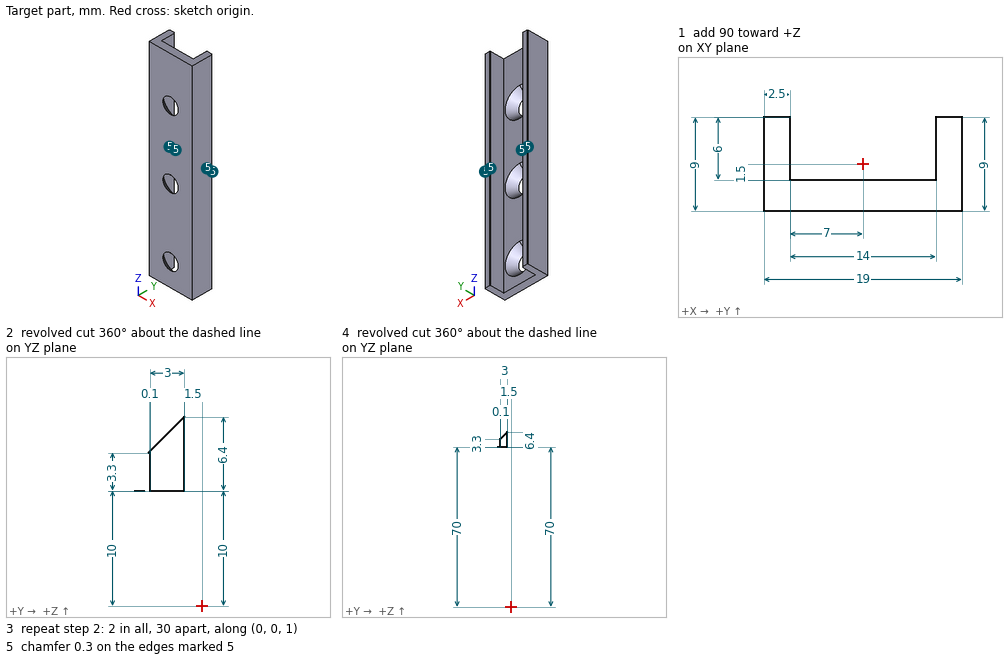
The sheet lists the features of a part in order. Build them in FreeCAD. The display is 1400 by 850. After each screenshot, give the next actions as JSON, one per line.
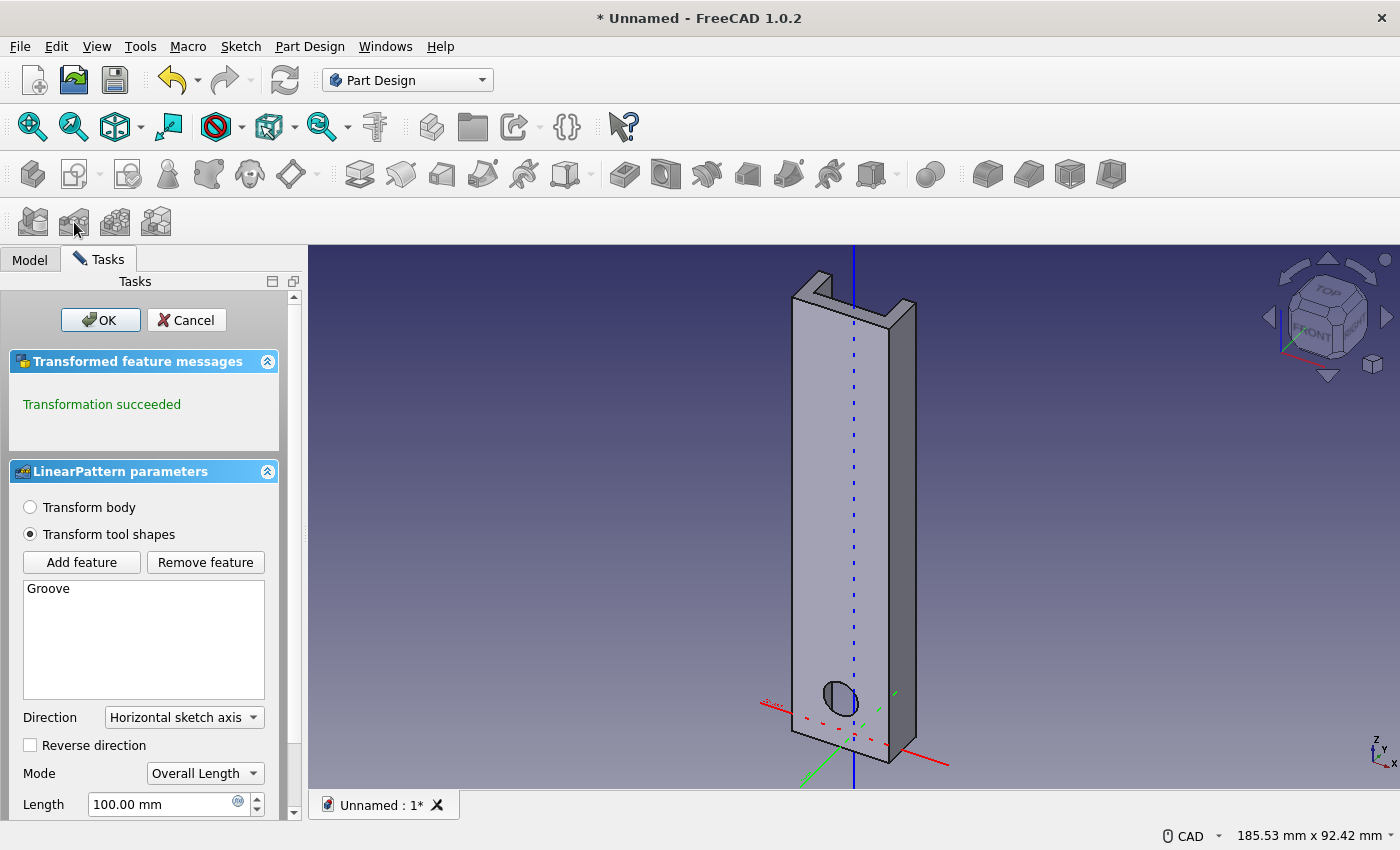
{"action": "left_click", "coordinate": [185, 718]}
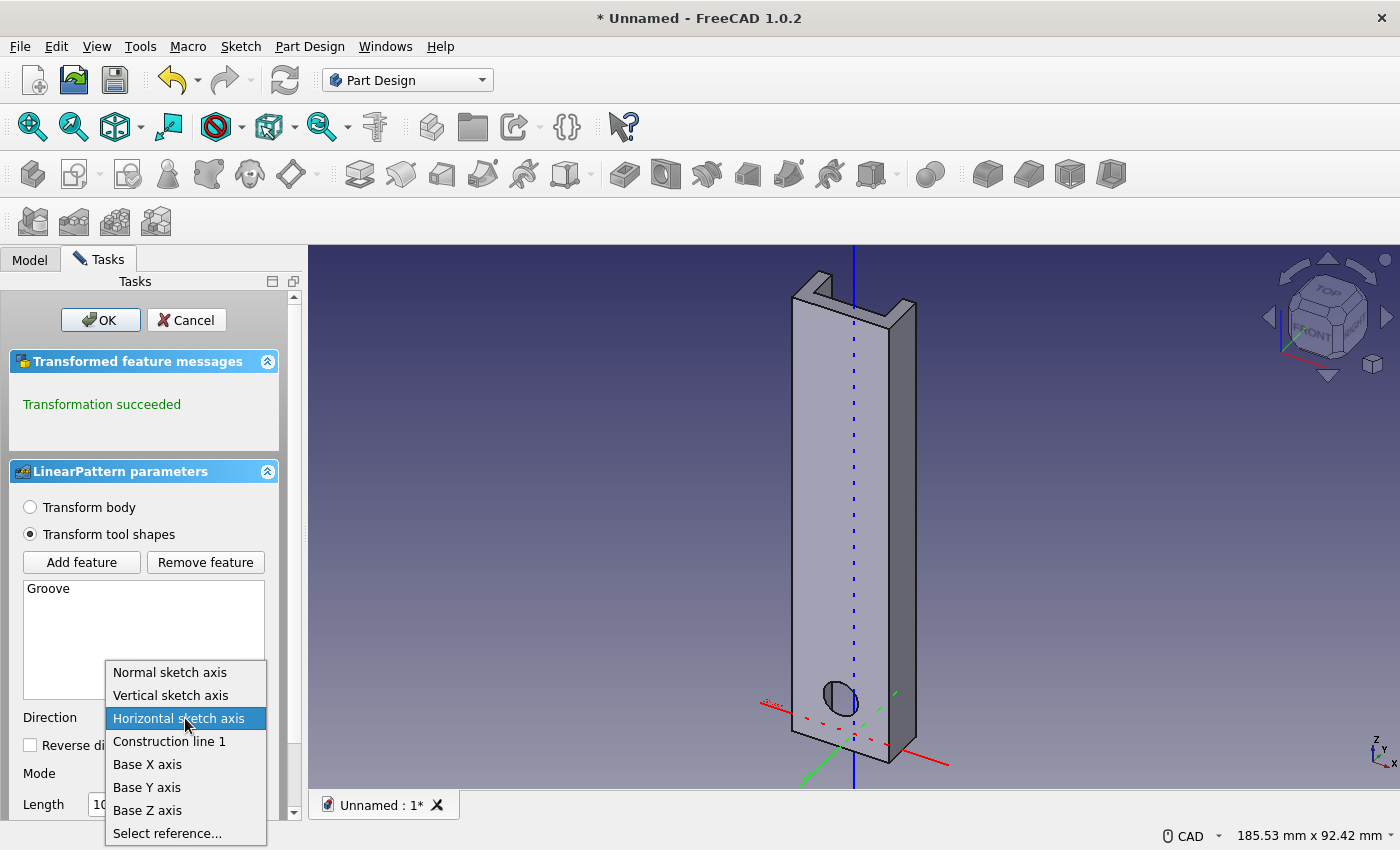
{"action": "left_click", "coordinate": [184, 810]}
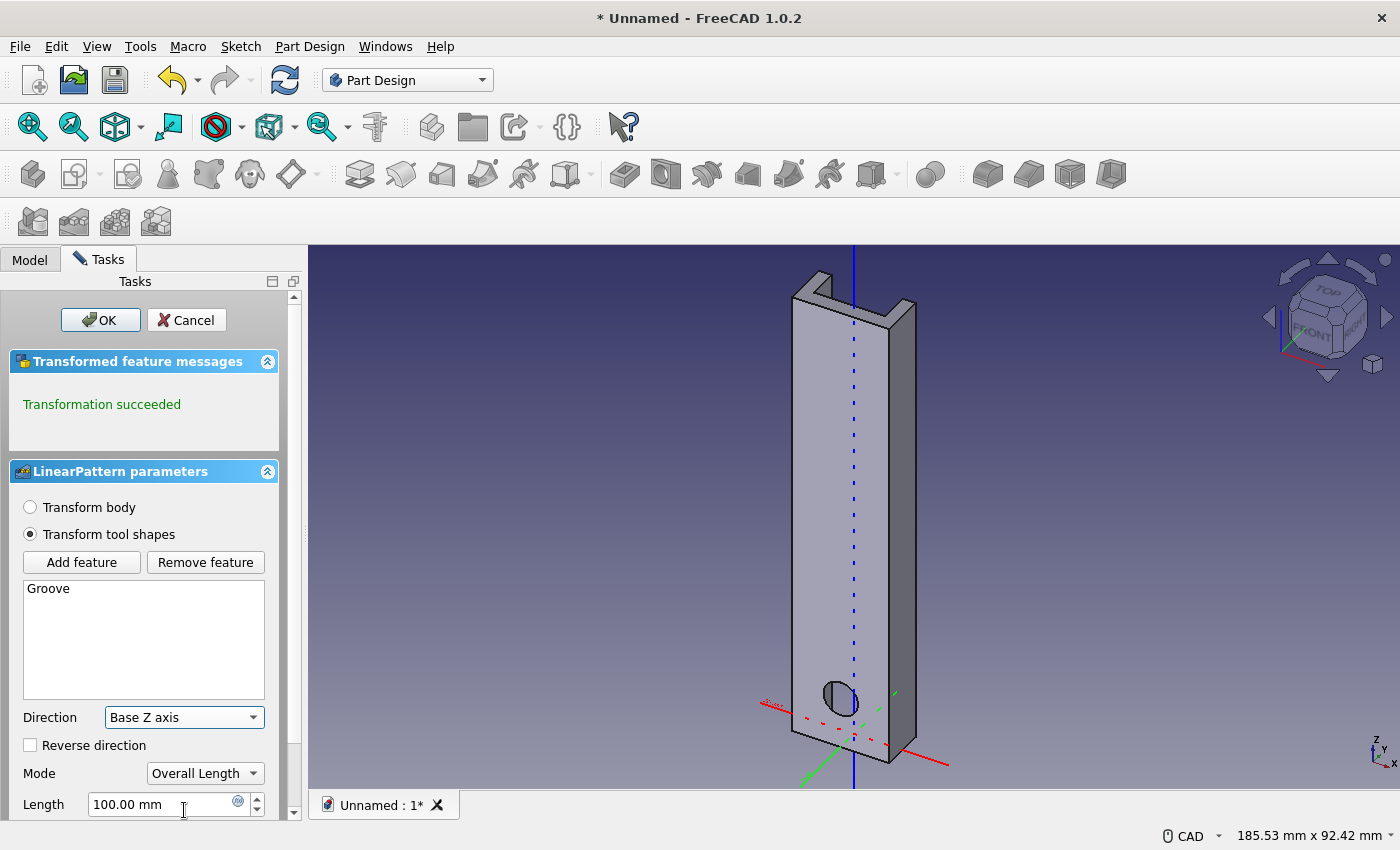
{"action": "left_click", "coordinate": [206, 774]}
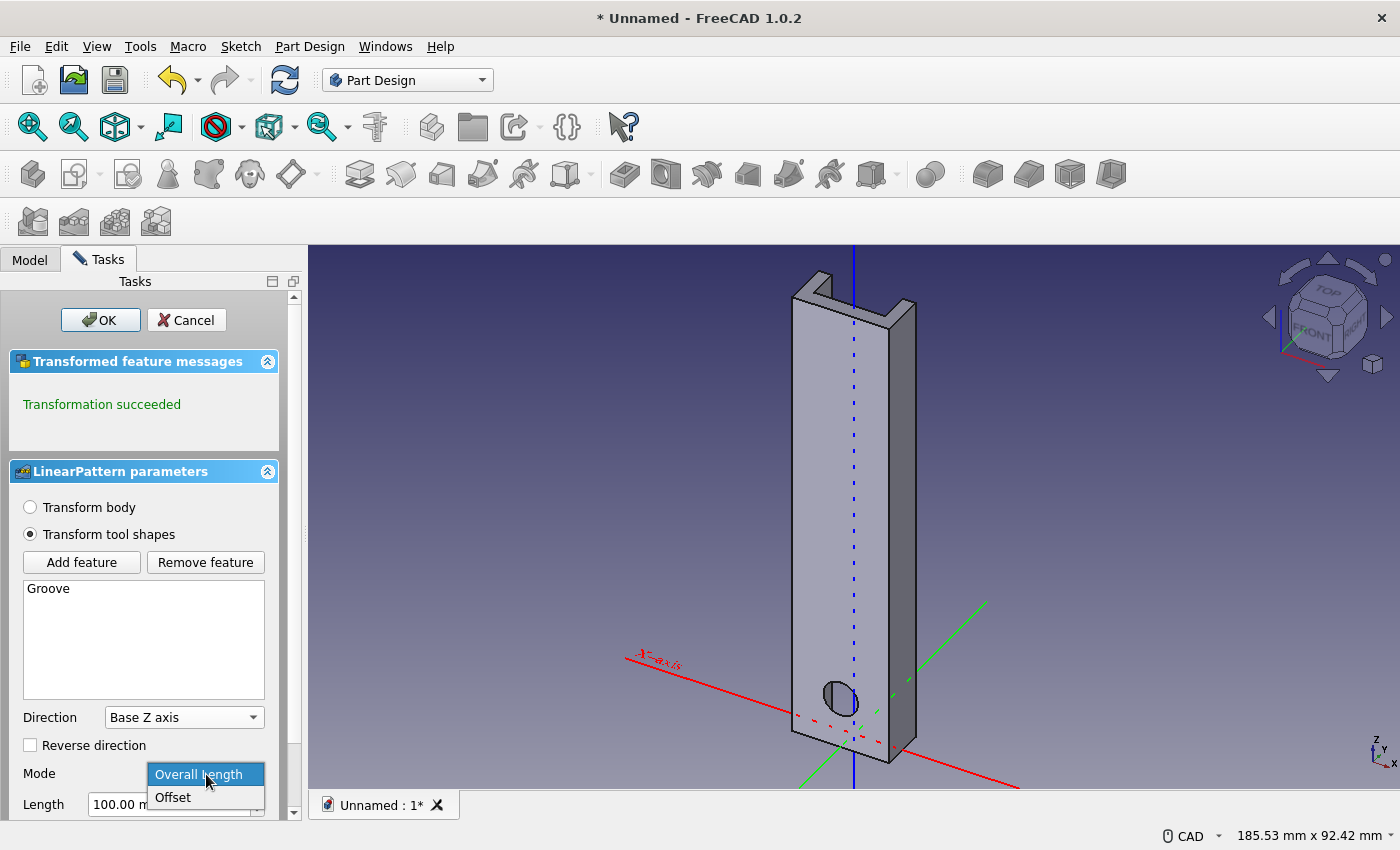
{"action": "left_click", "coordinate": [204, 798]}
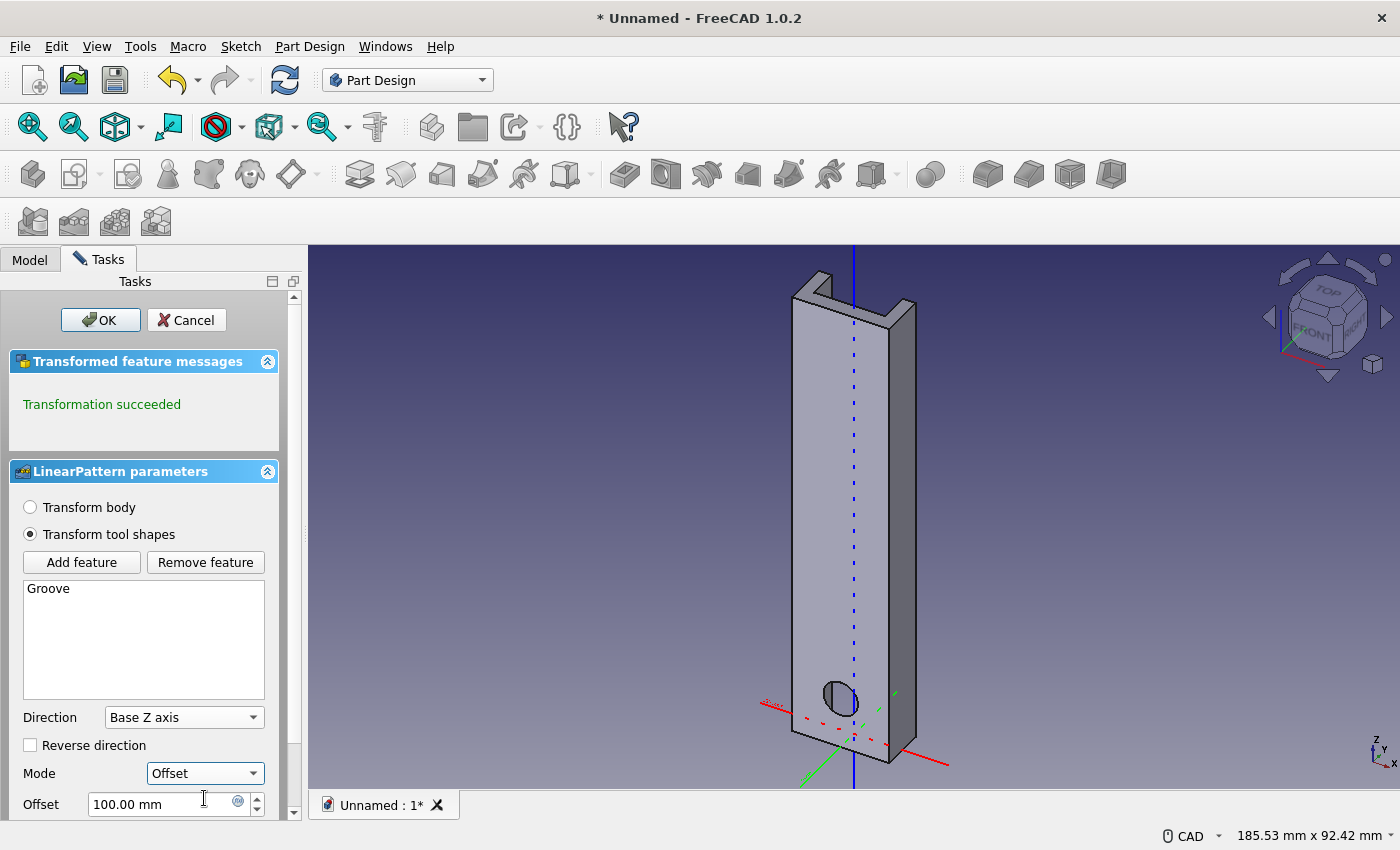
{"action": "triple_click", "coordinate": [170, 804]}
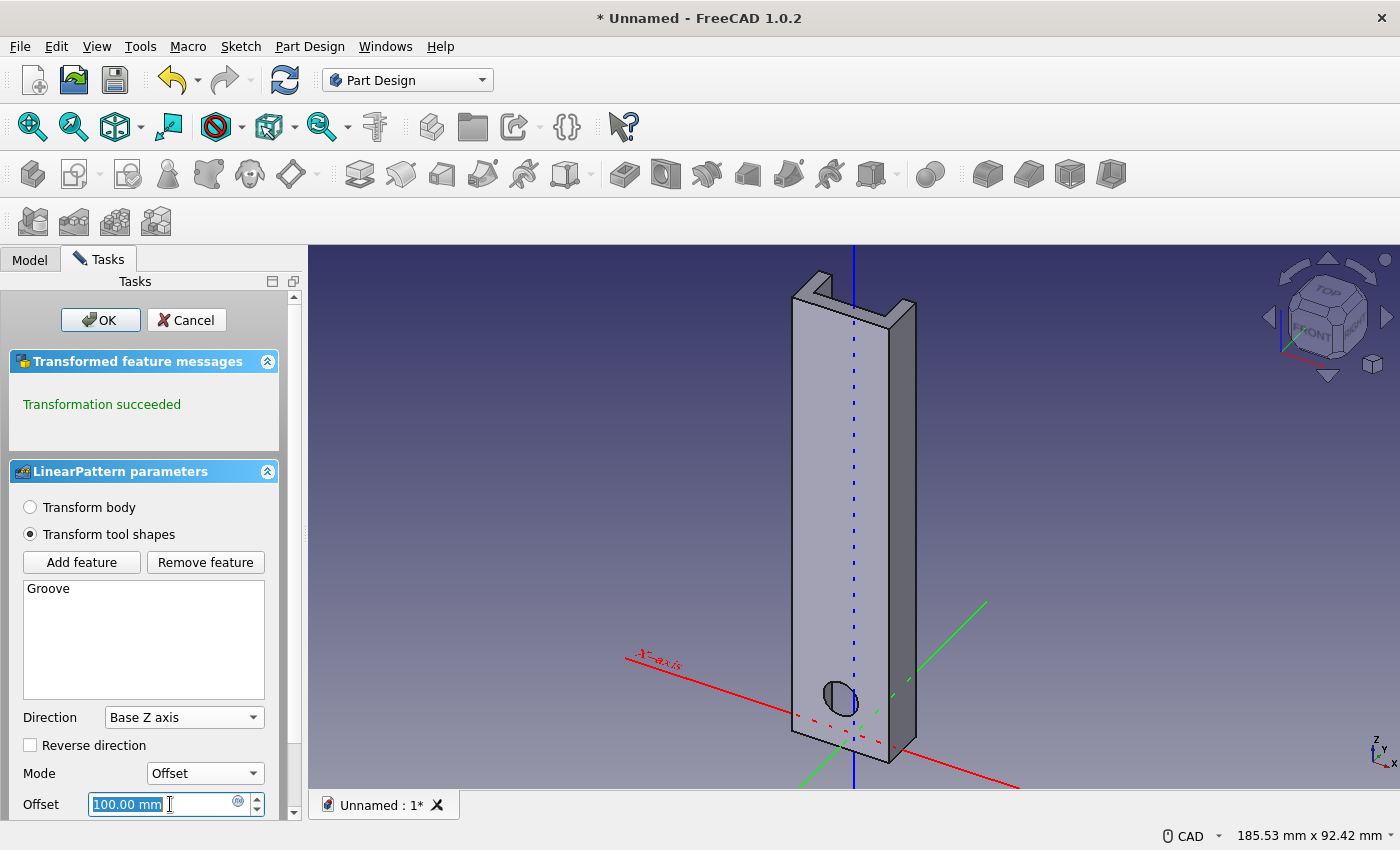
{"action": "type", "text": "30"}
{"action": "key", "text": "Tab"}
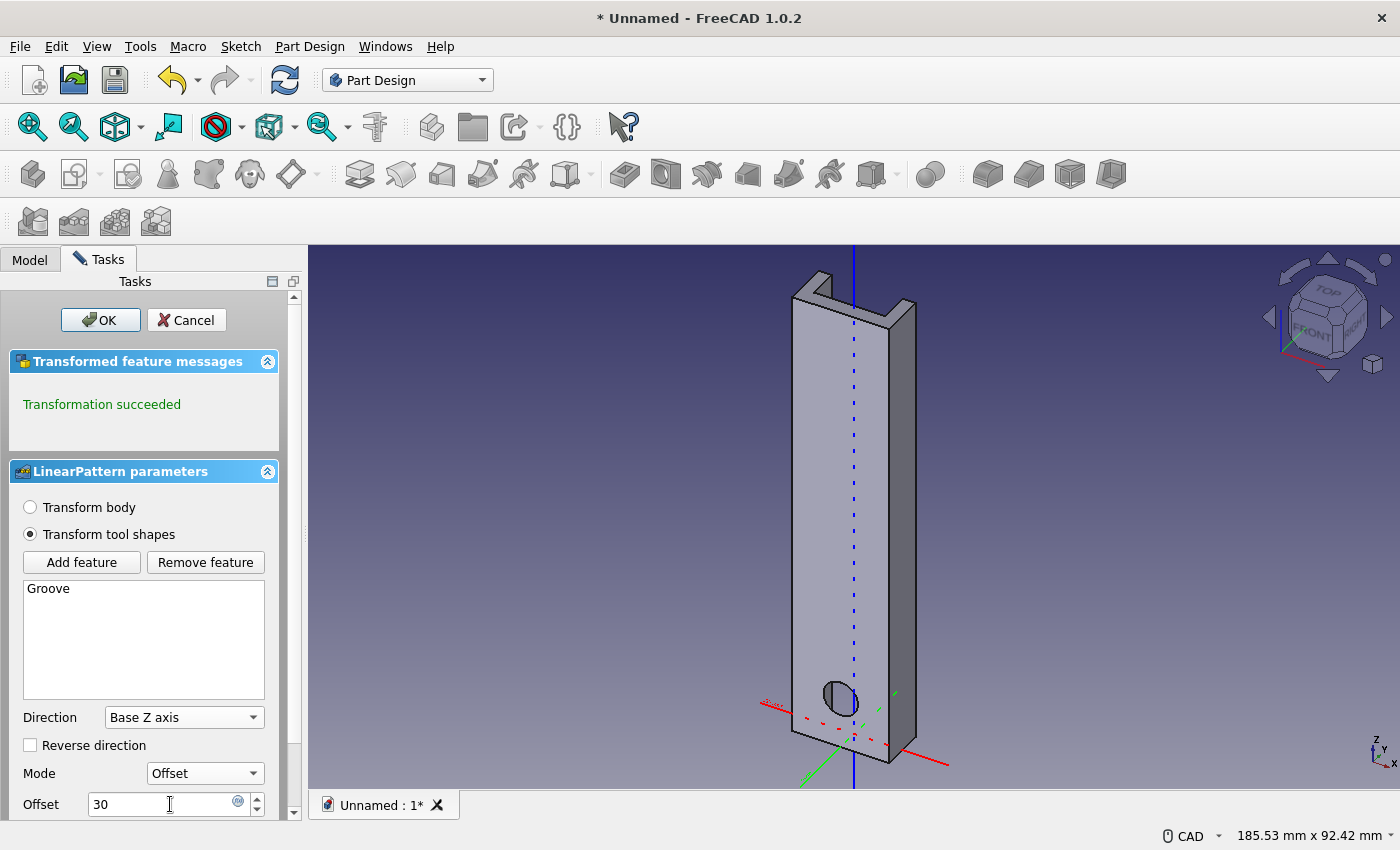
{"action": "scroll", "coordinate": [294, 556], "scroll_direction": "down", "scroll_amount": 2}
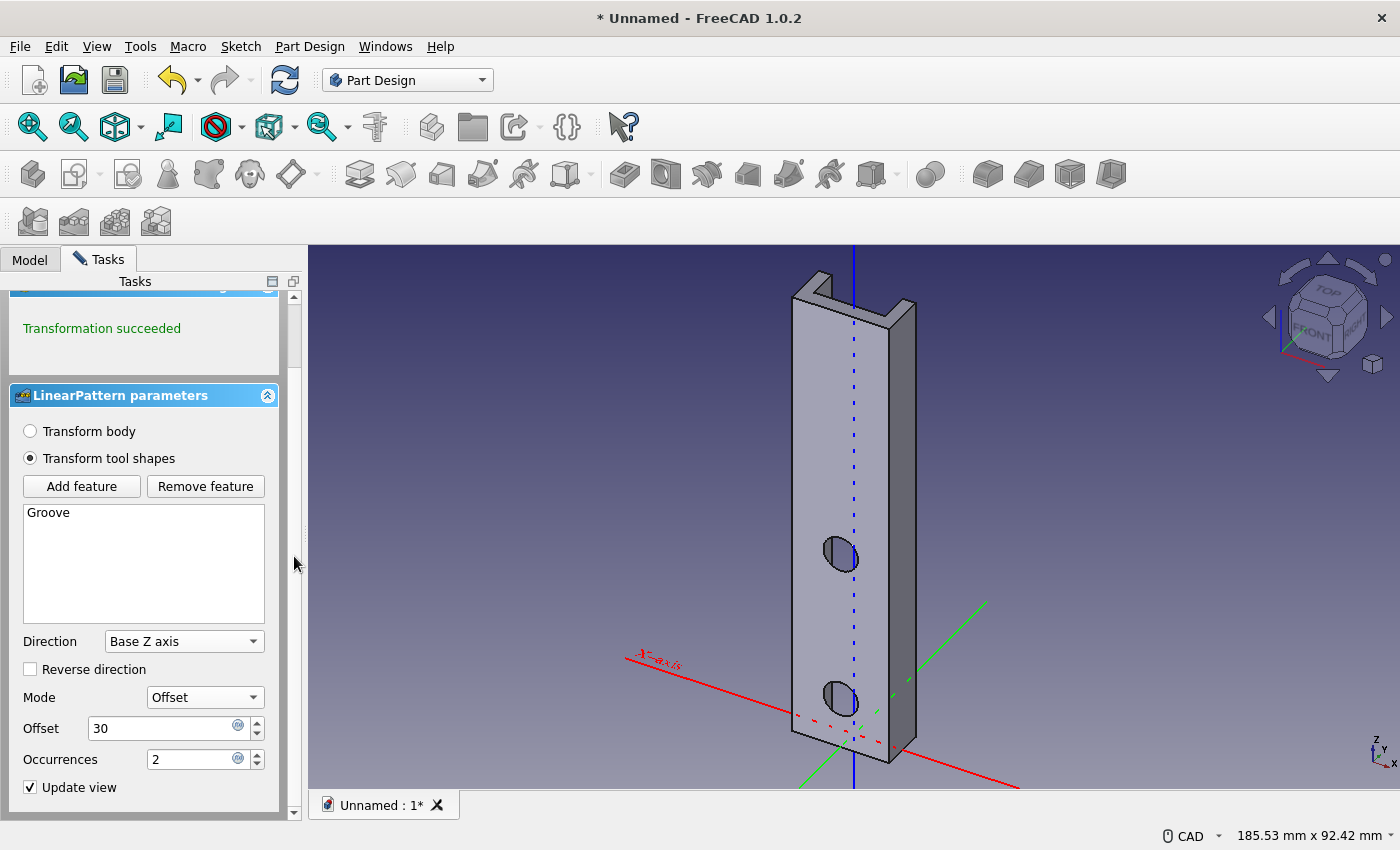
{"action": "triple_click", "coordinate": [199, 760]}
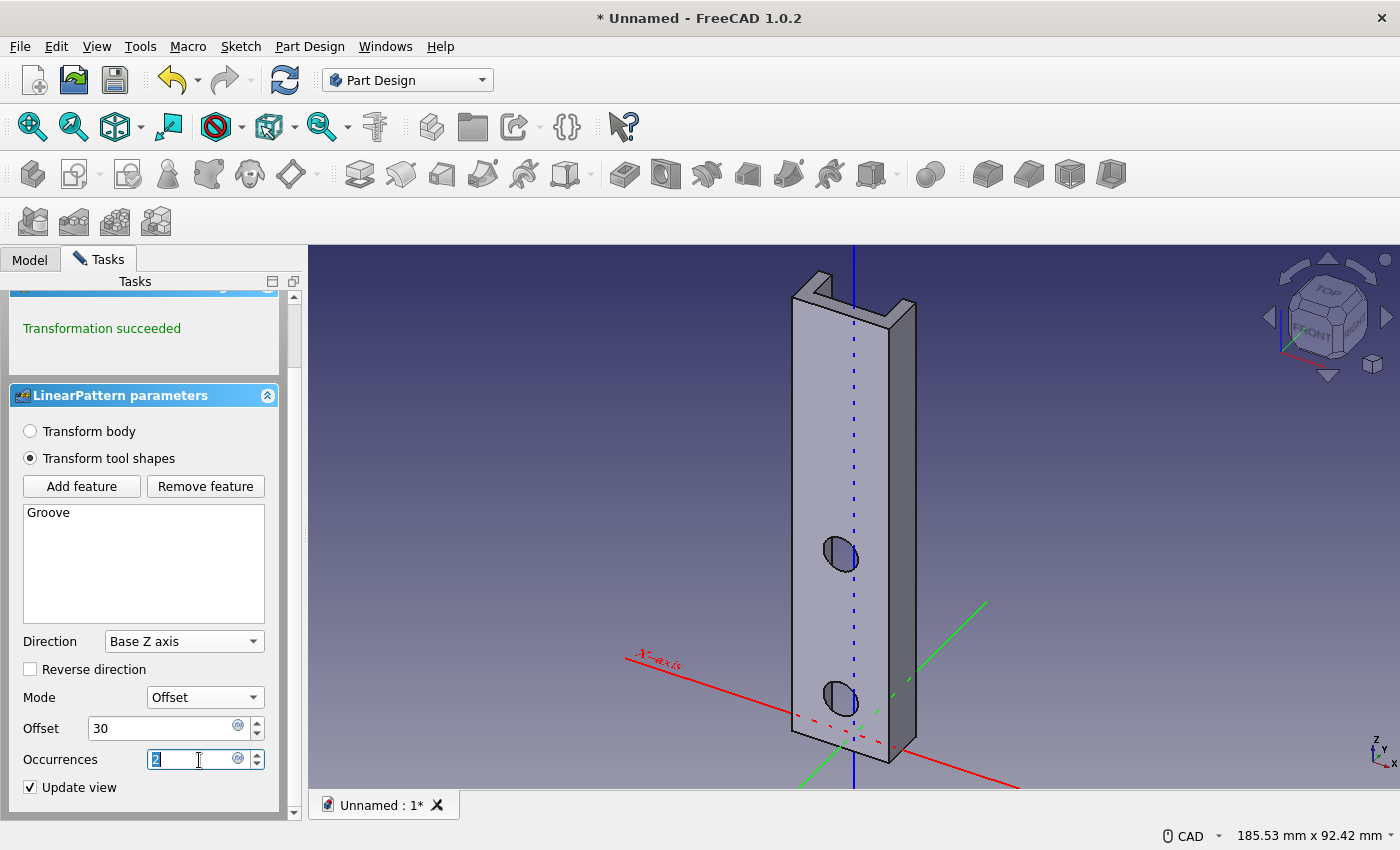
{"action": "type", "text": "2"}
{"action": "key", "text": "Tab"}